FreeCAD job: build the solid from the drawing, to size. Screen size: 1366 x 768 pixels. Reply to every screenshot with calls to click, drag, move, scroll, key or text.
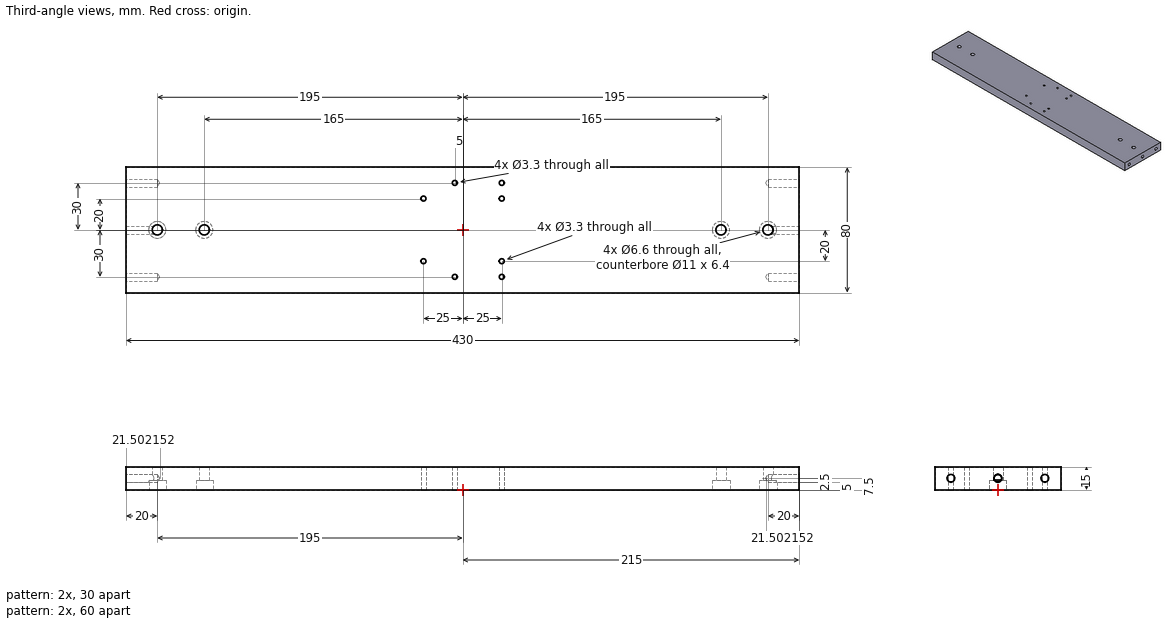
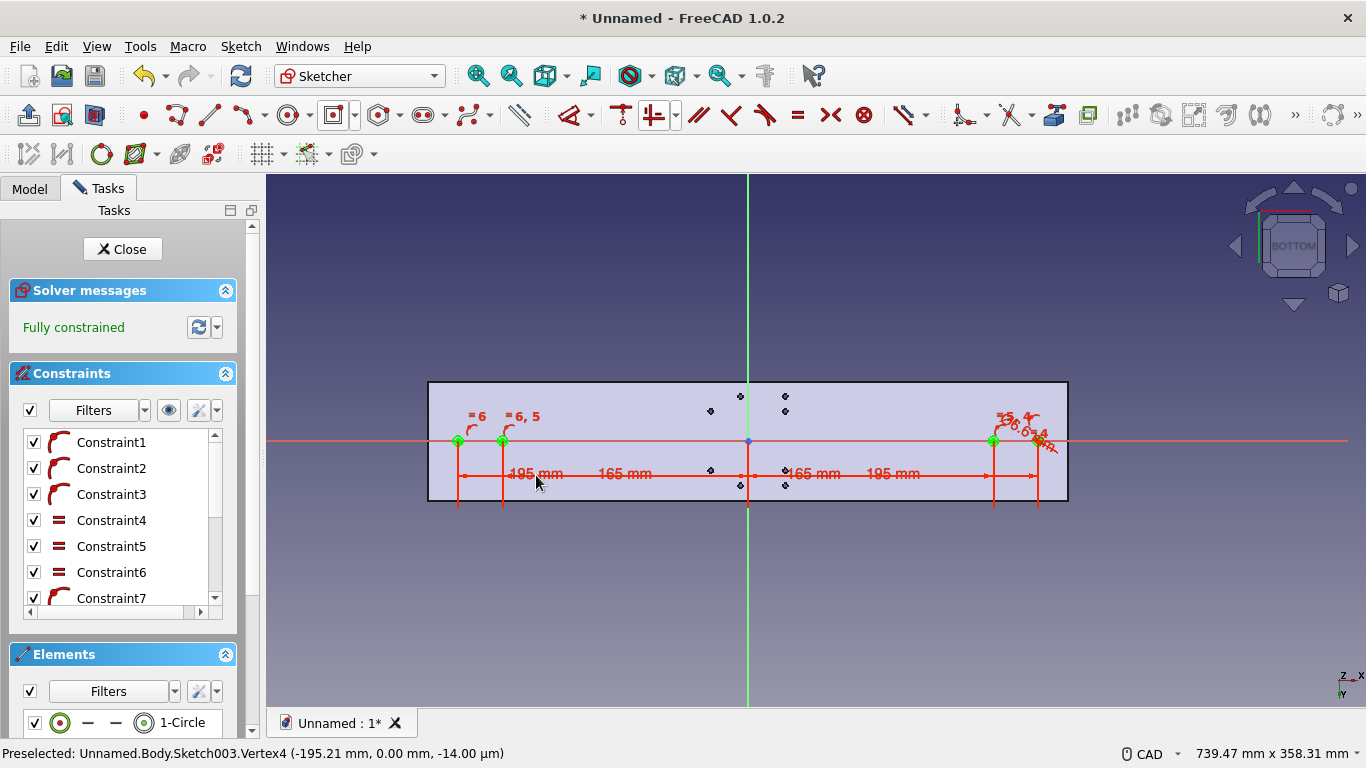
click(123, 249)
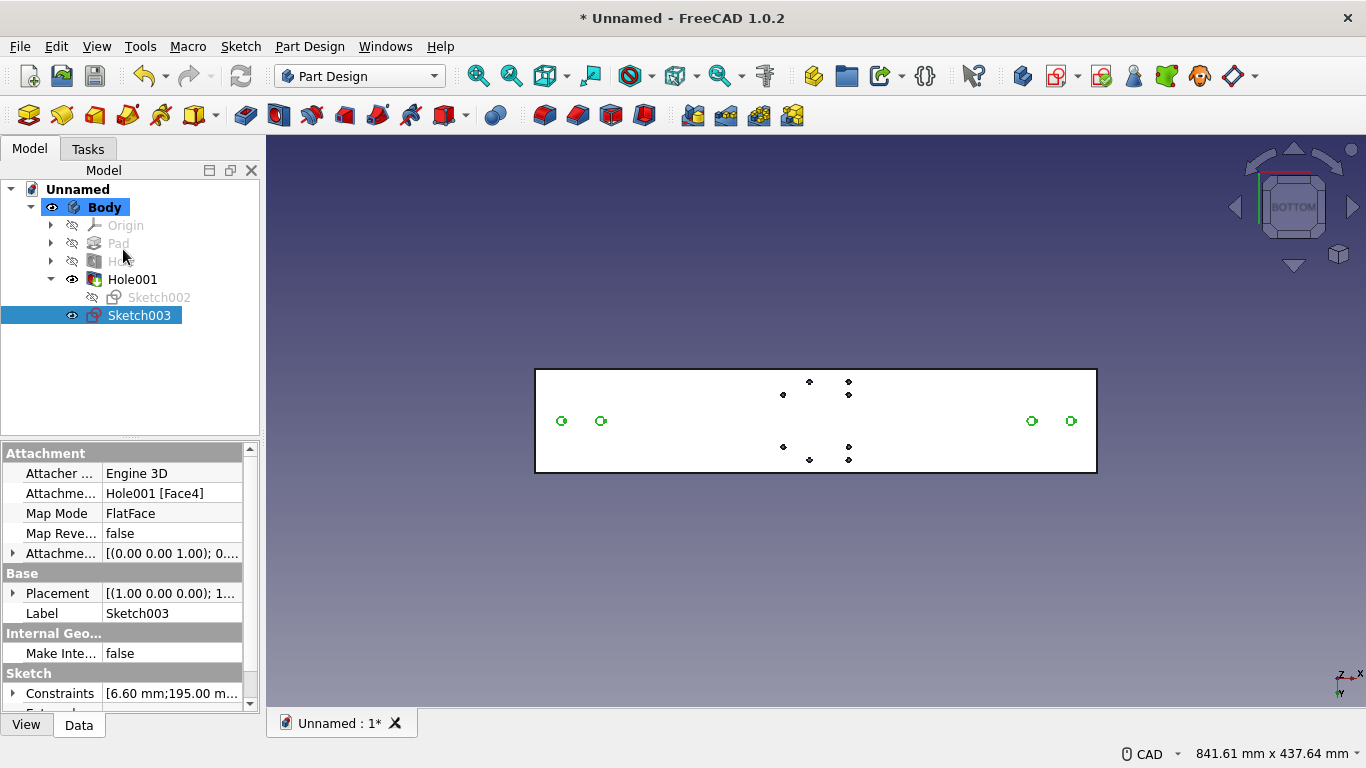
click(279, 116)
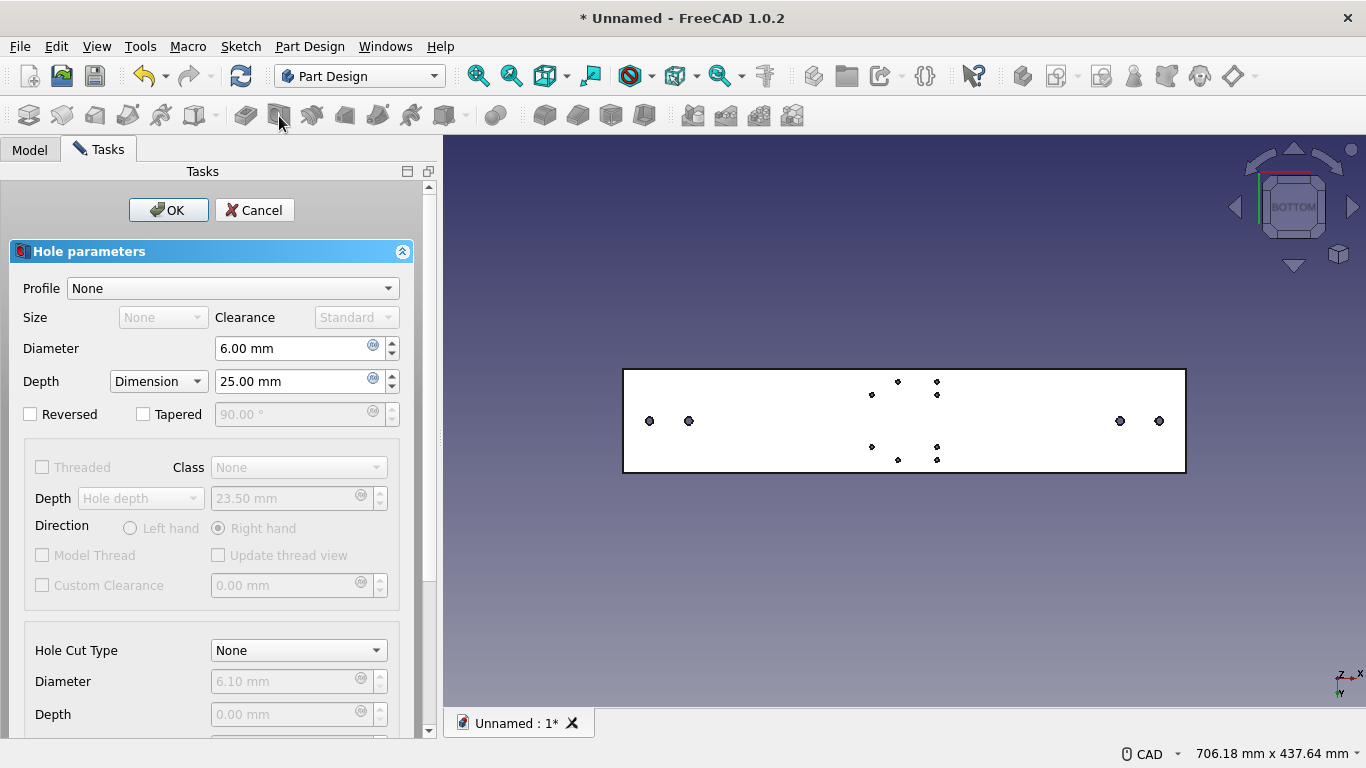
triple_click(300, 348)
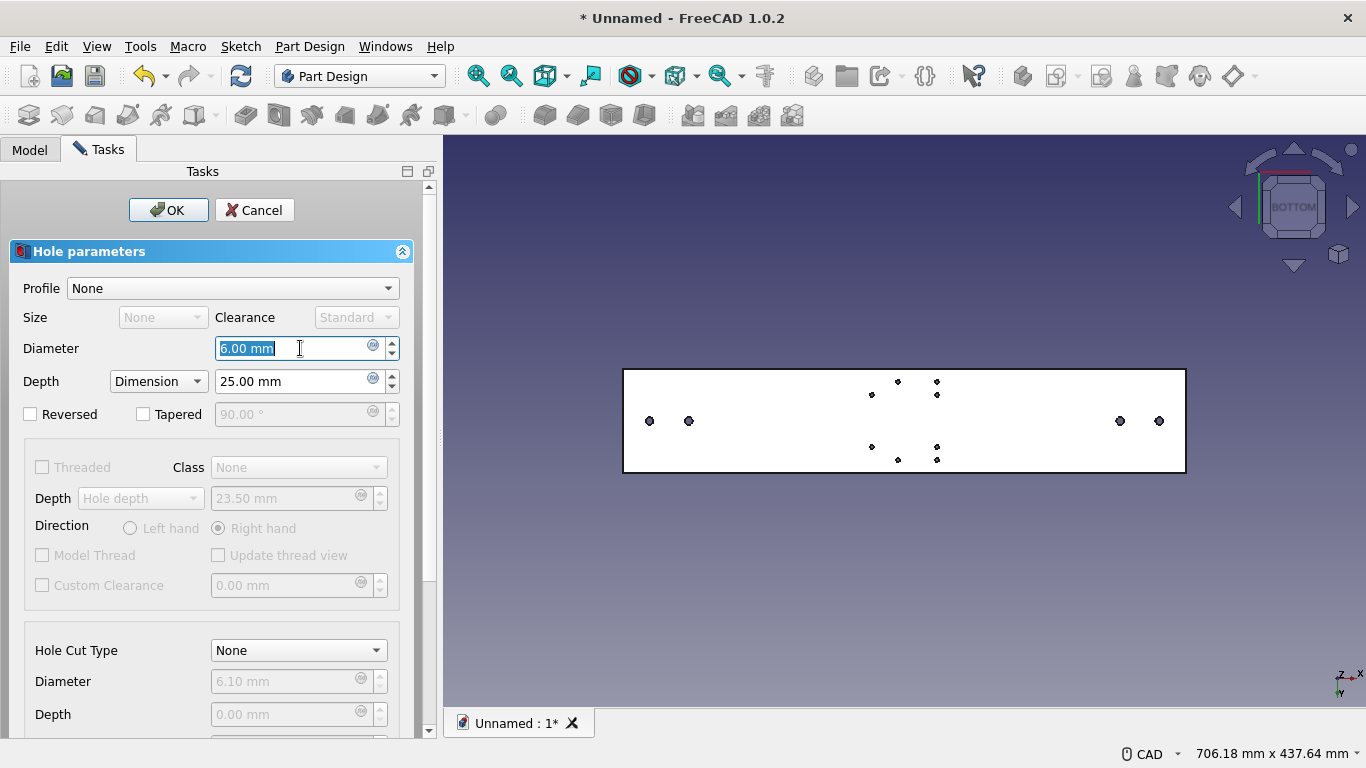
text(6.6)
key(Tab)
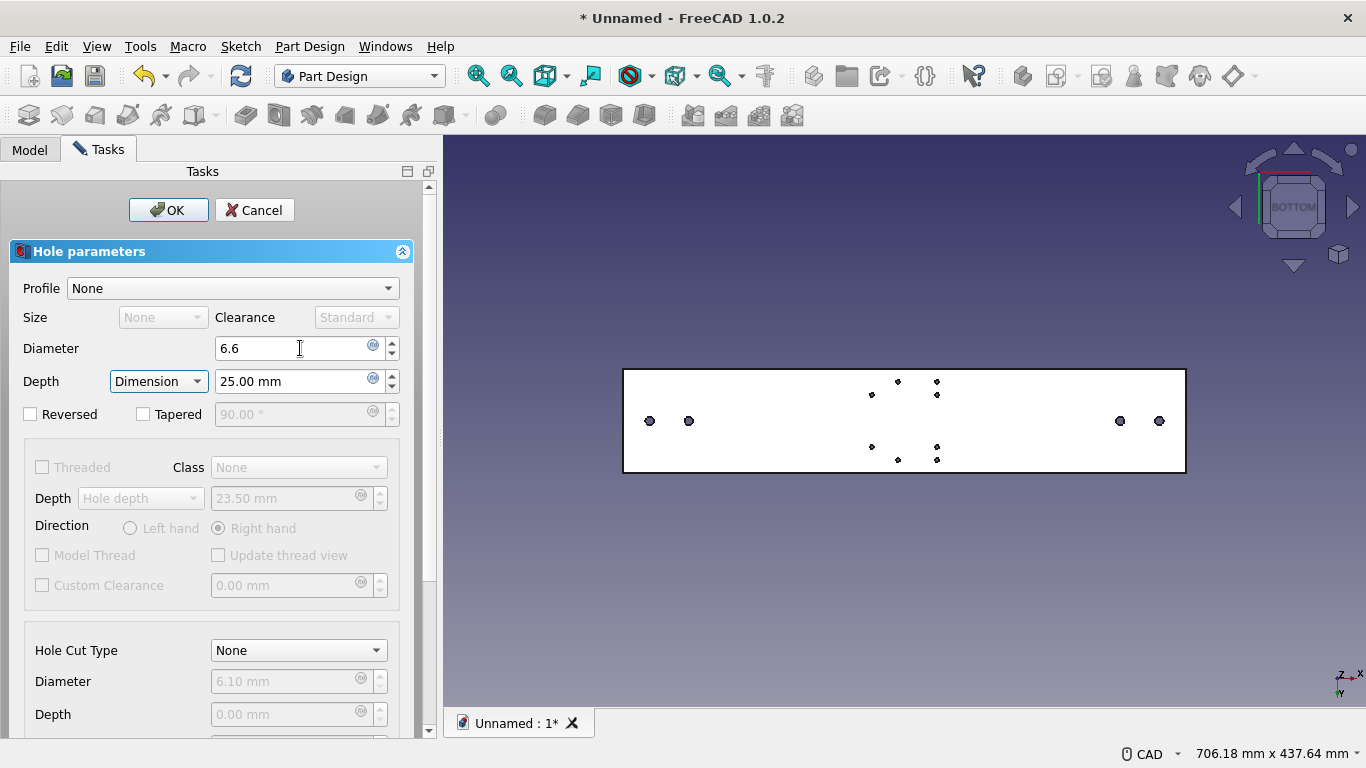
click(160, 382)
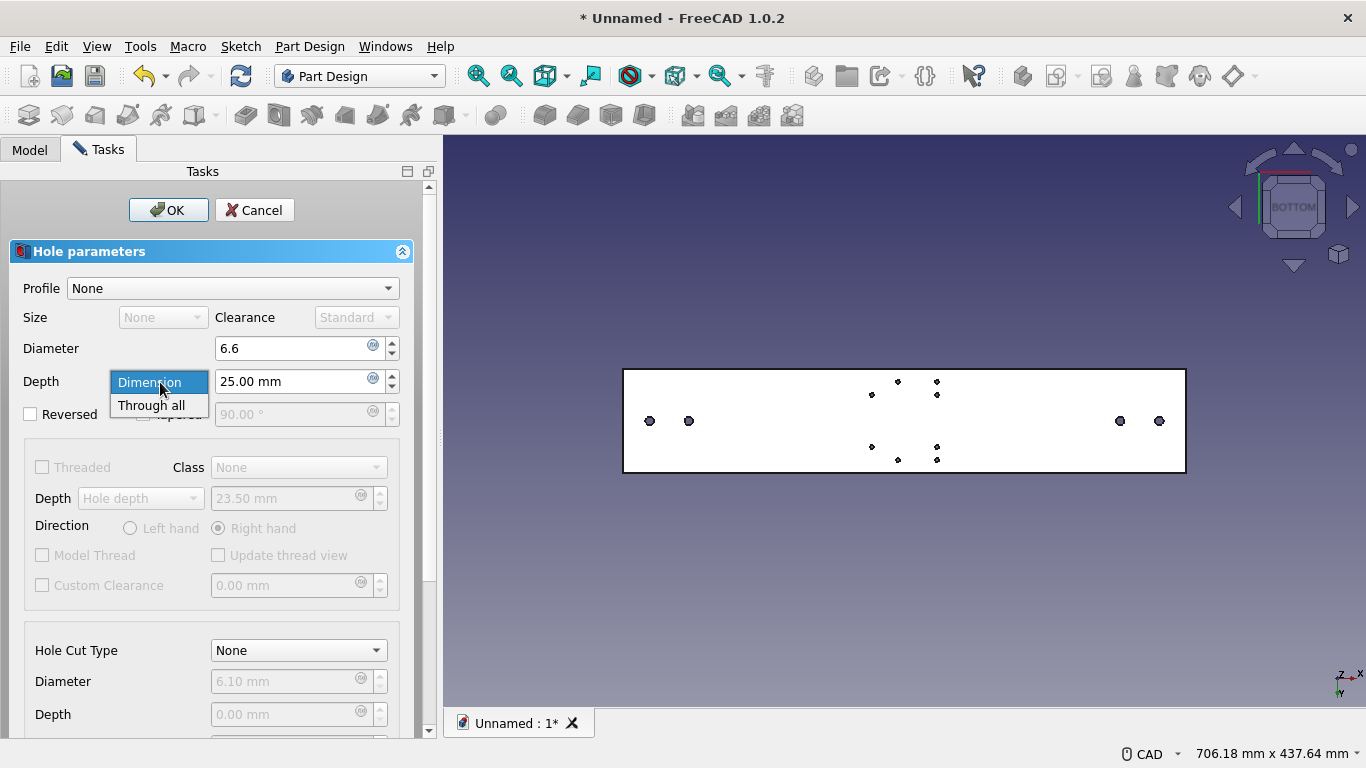
click(158, 406)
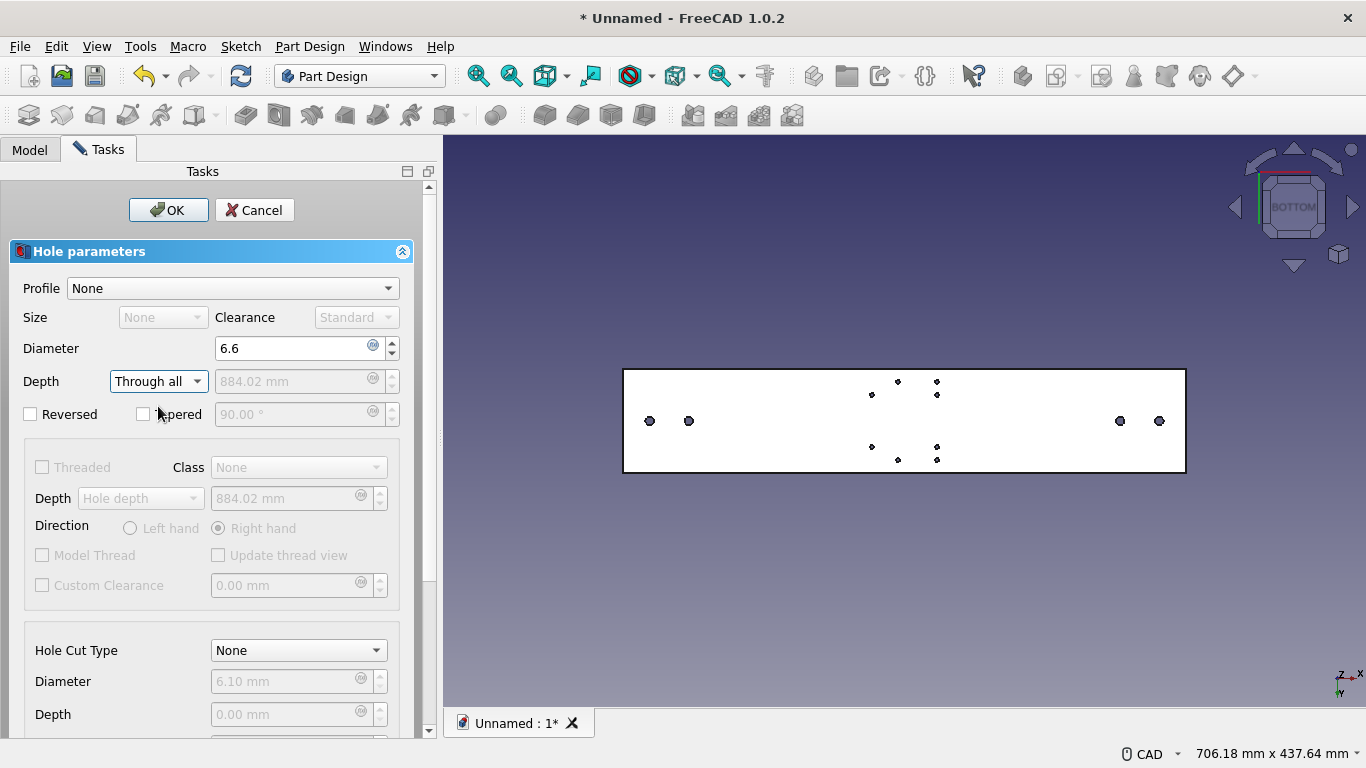
click(300, 650)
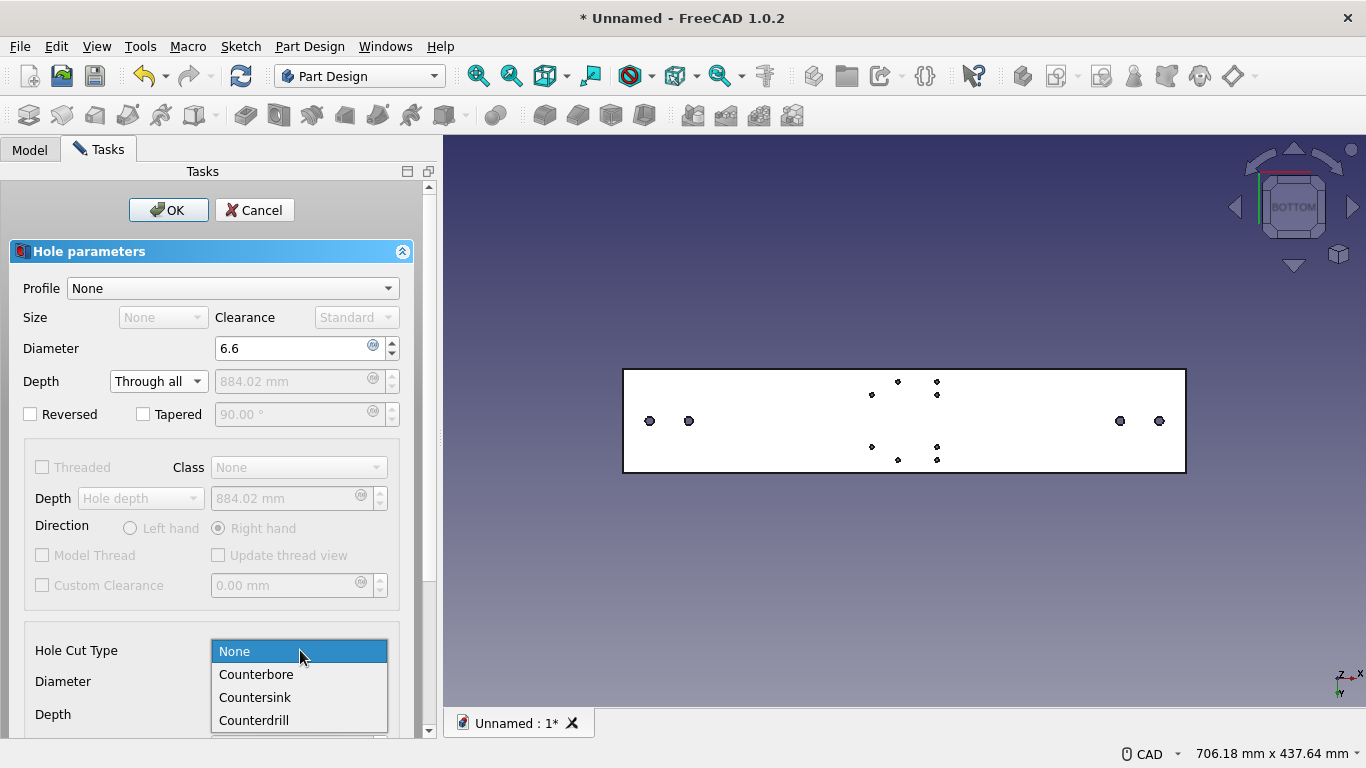
click(298, 674)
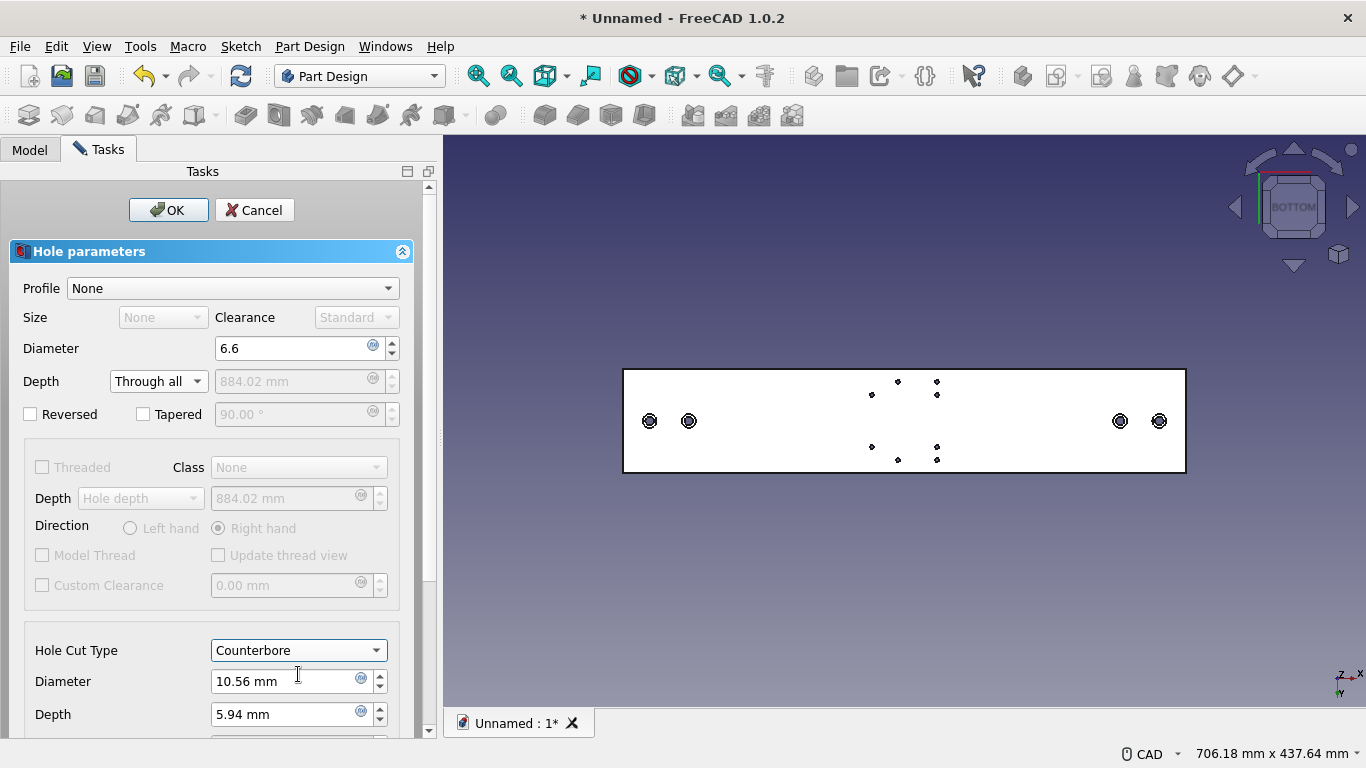
triple_click(292, 682)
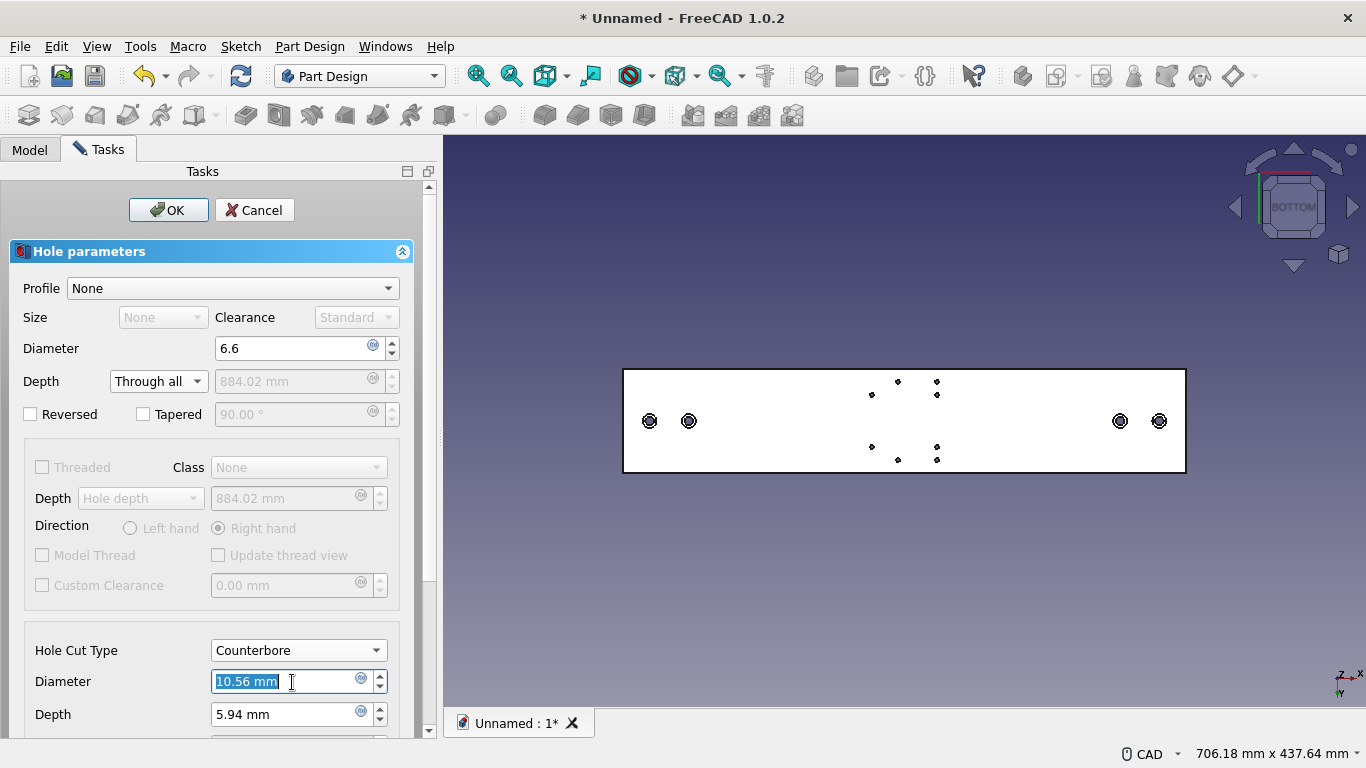
text(11)
key(Tab)